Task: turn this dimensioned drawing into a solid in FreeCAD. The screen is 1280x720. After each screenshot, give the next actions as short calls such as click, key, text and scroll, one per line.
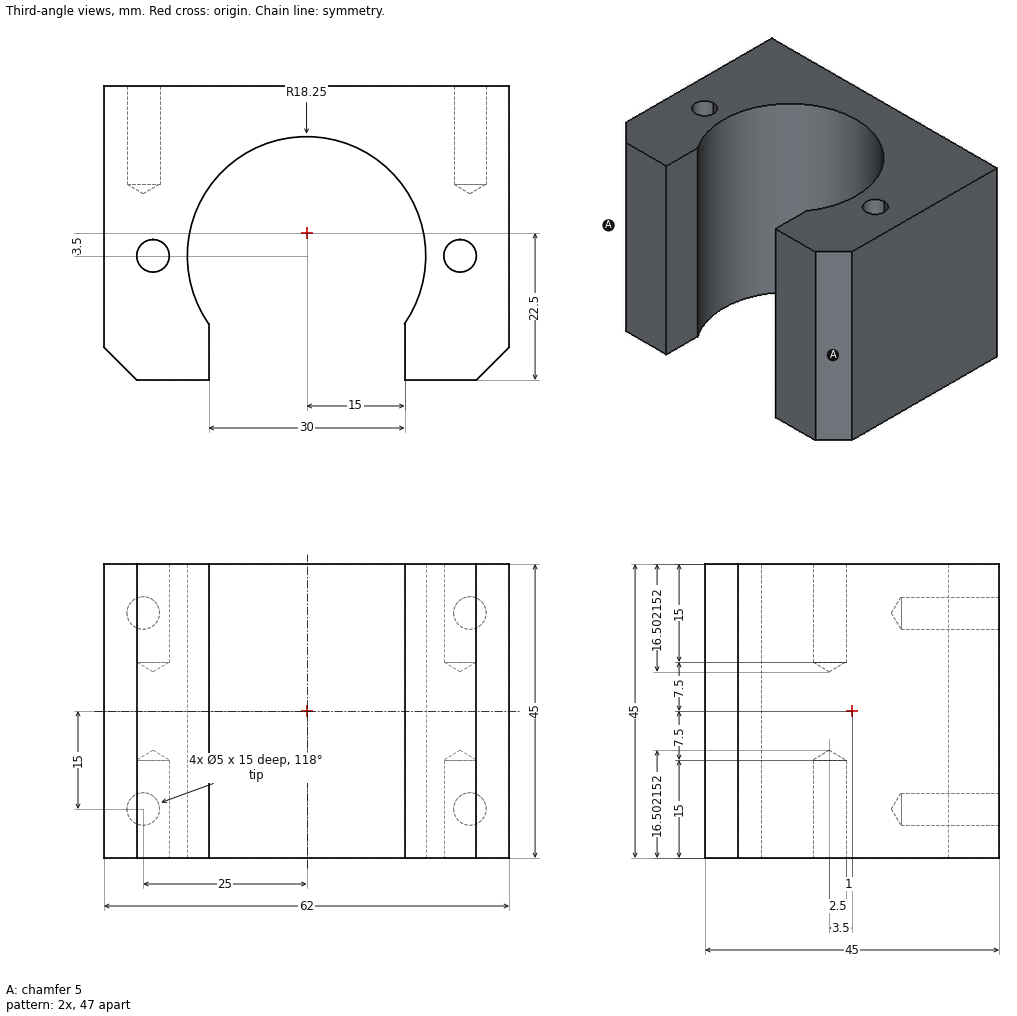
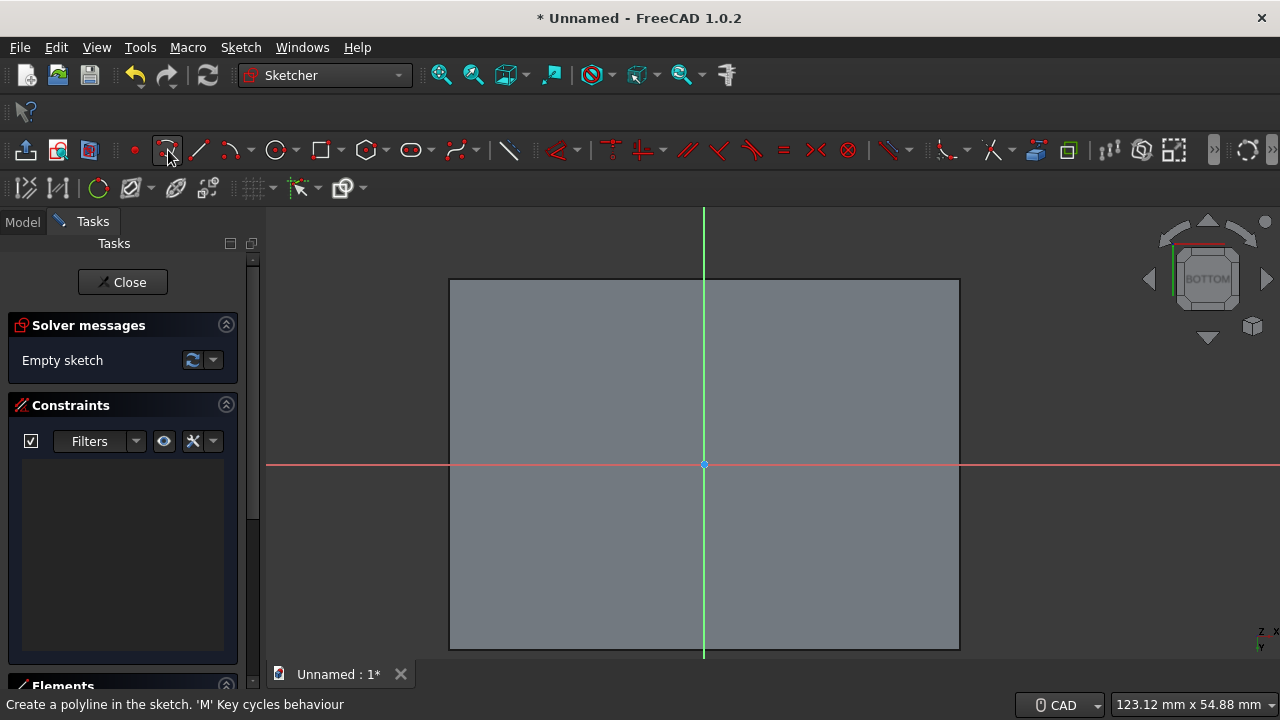
click(828, 350)
click(828, 279)
click(581, 279)
click(581, 350)
right_click(581, 350)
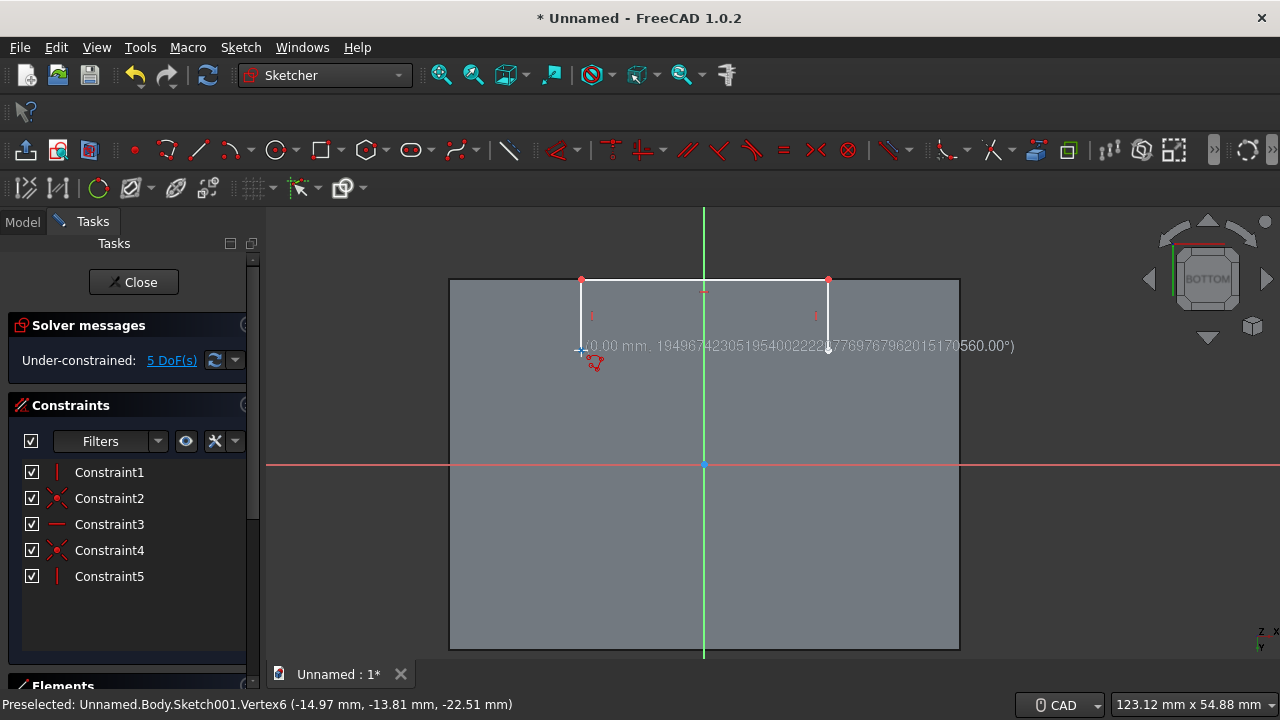
key(g)
key(3)
key(a)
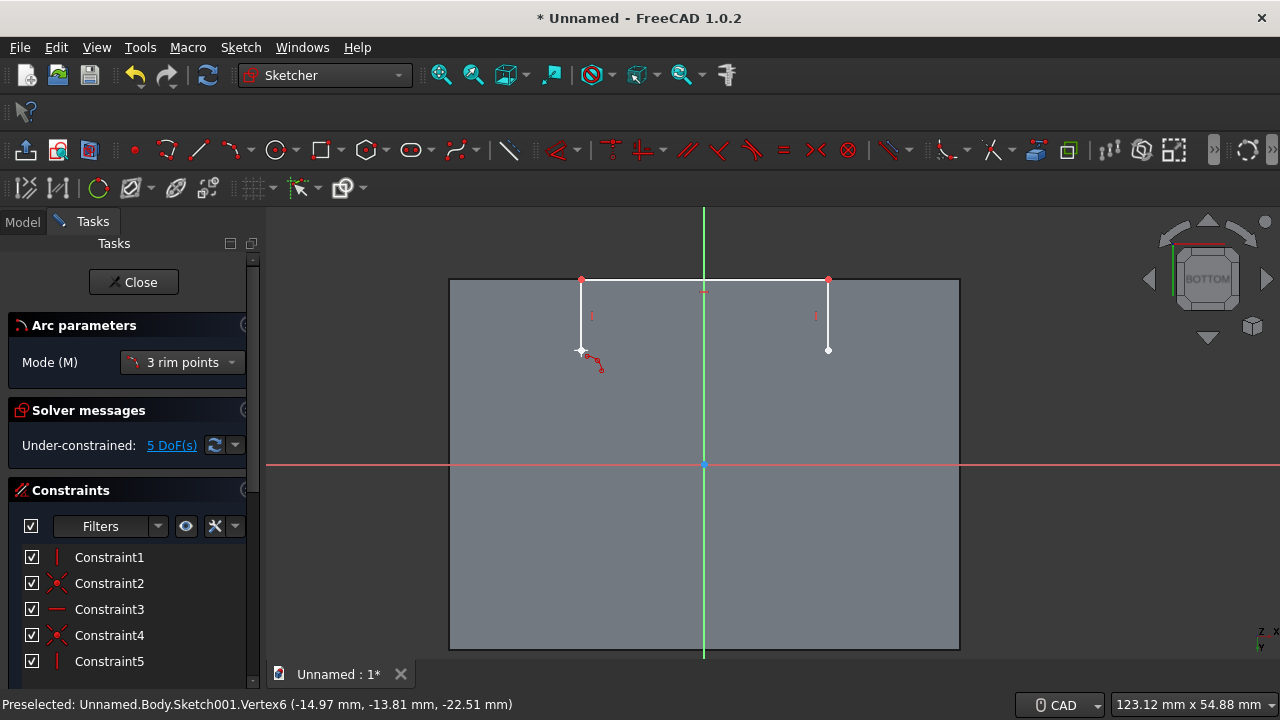
click(581, 351)
click(828, 351)
click(641, 572)
key(Escape)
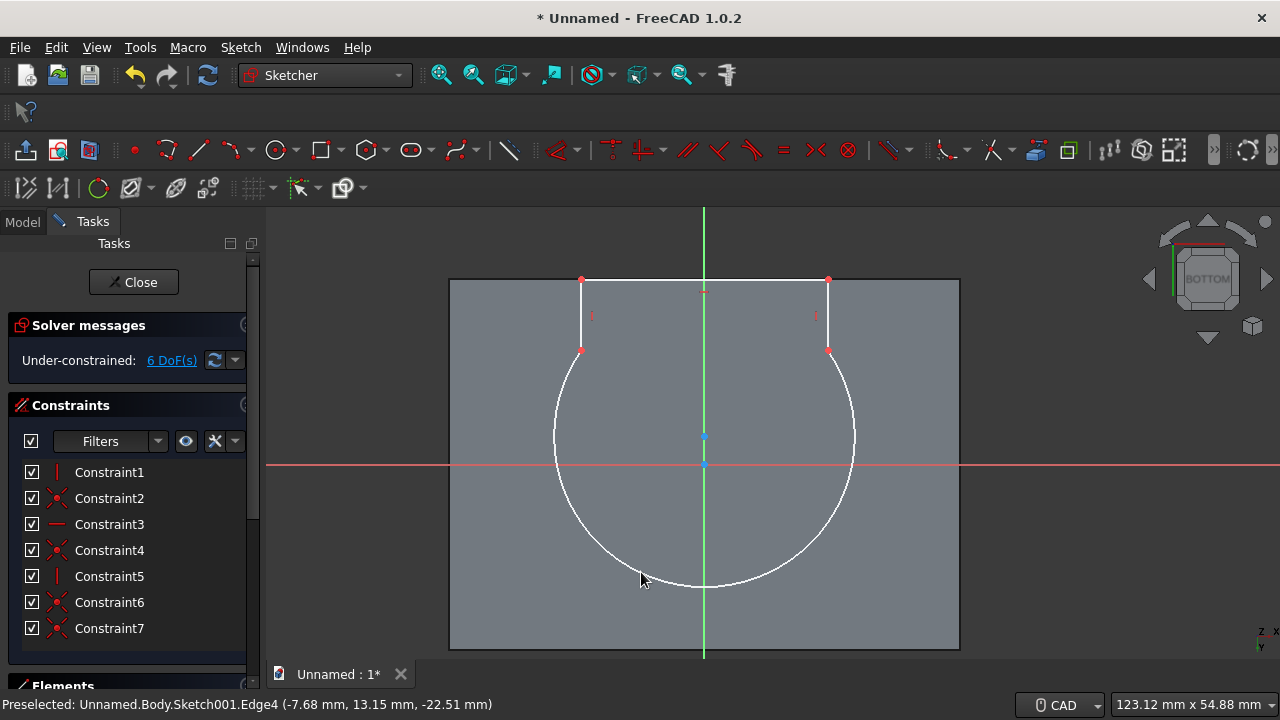
click(704, 437)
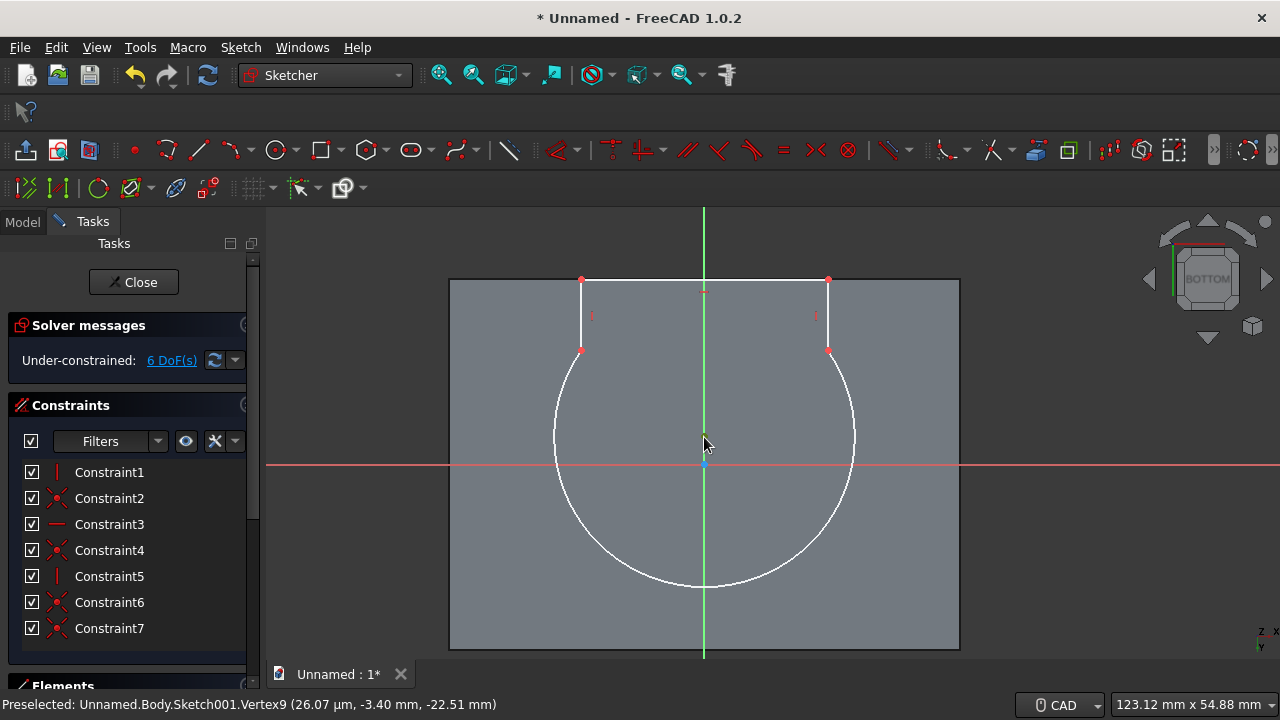
click(704, 546)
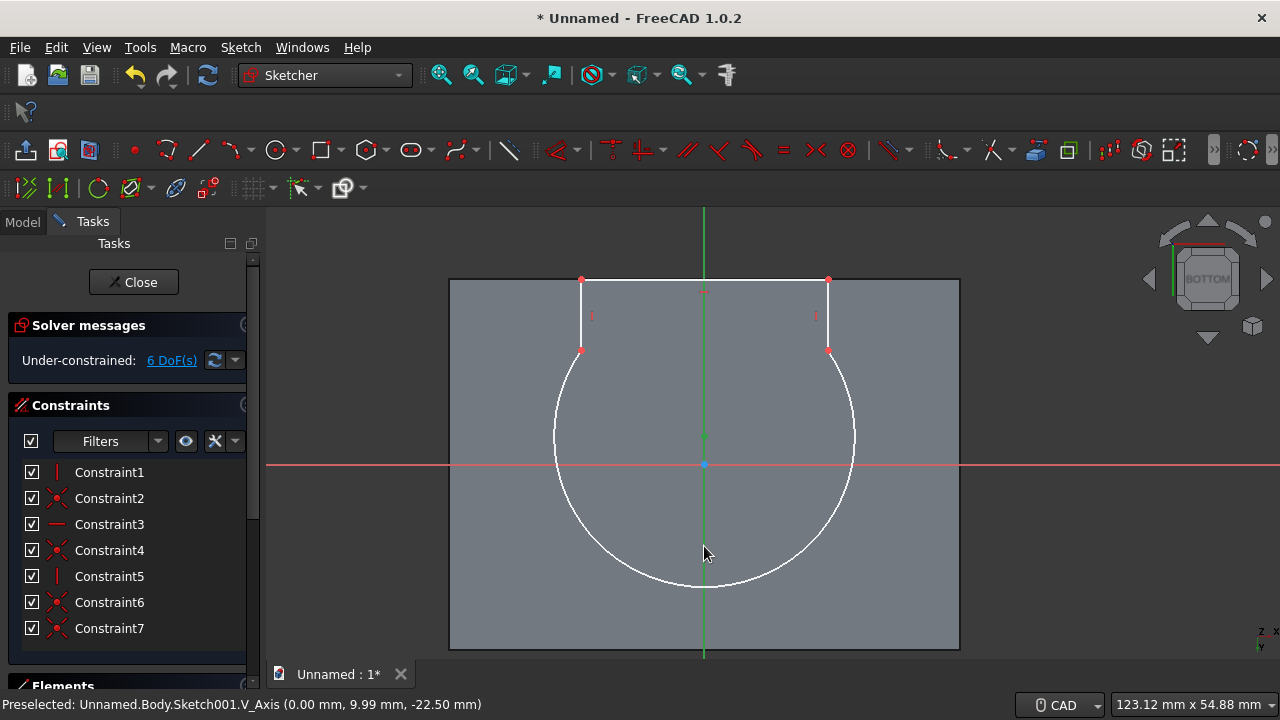
click(612, 150)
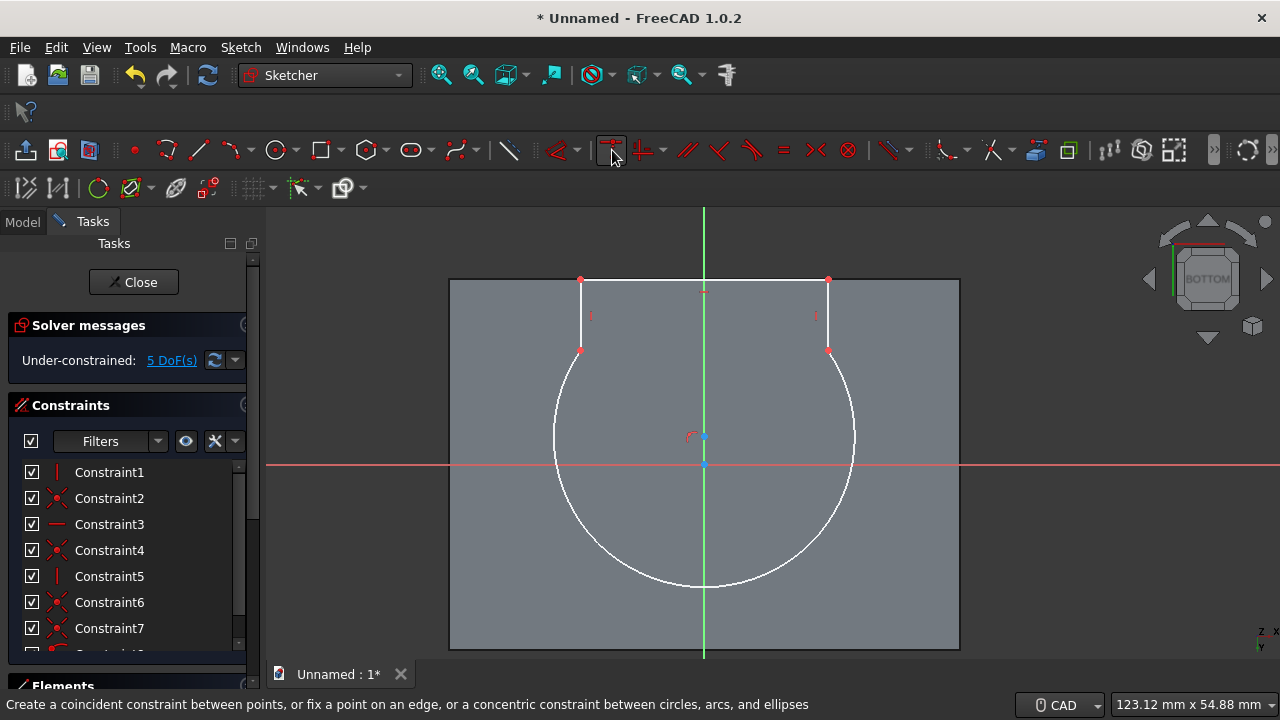
click(556, 150)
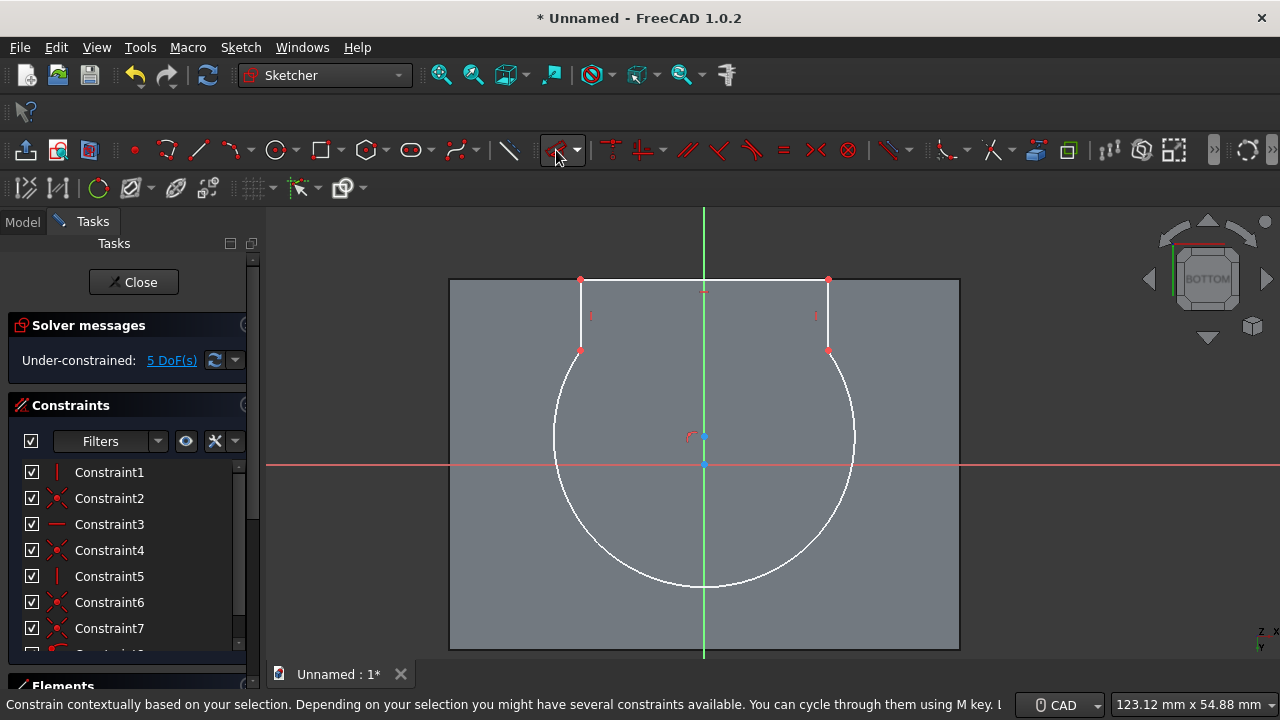
click(589, 534)
click(565, 555)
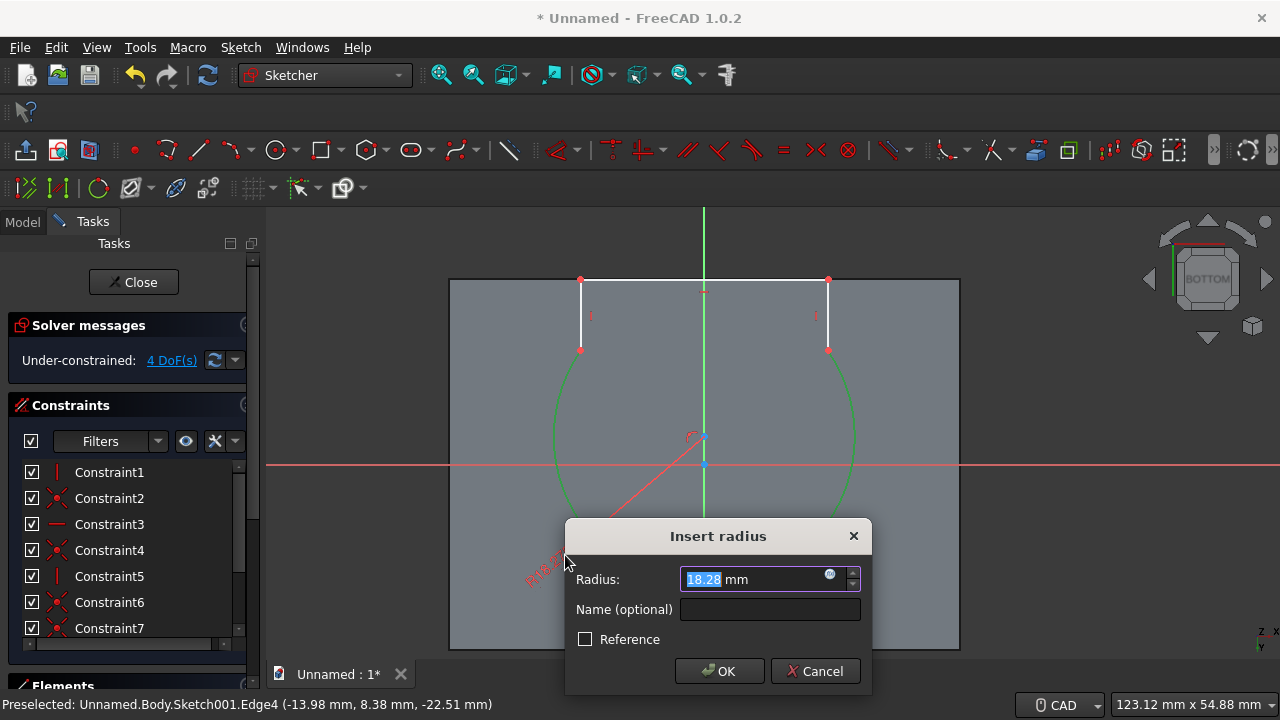
text(18.25)
key(Return)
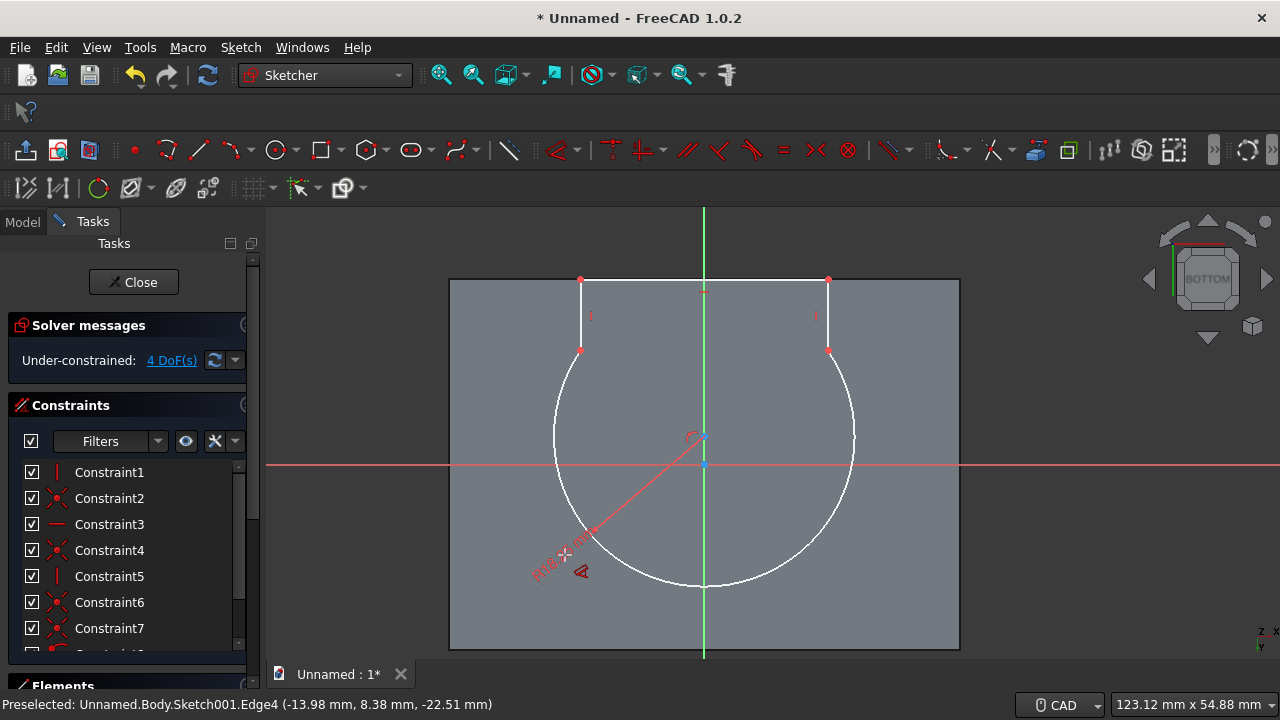
click(754, 280)
click(647, 246)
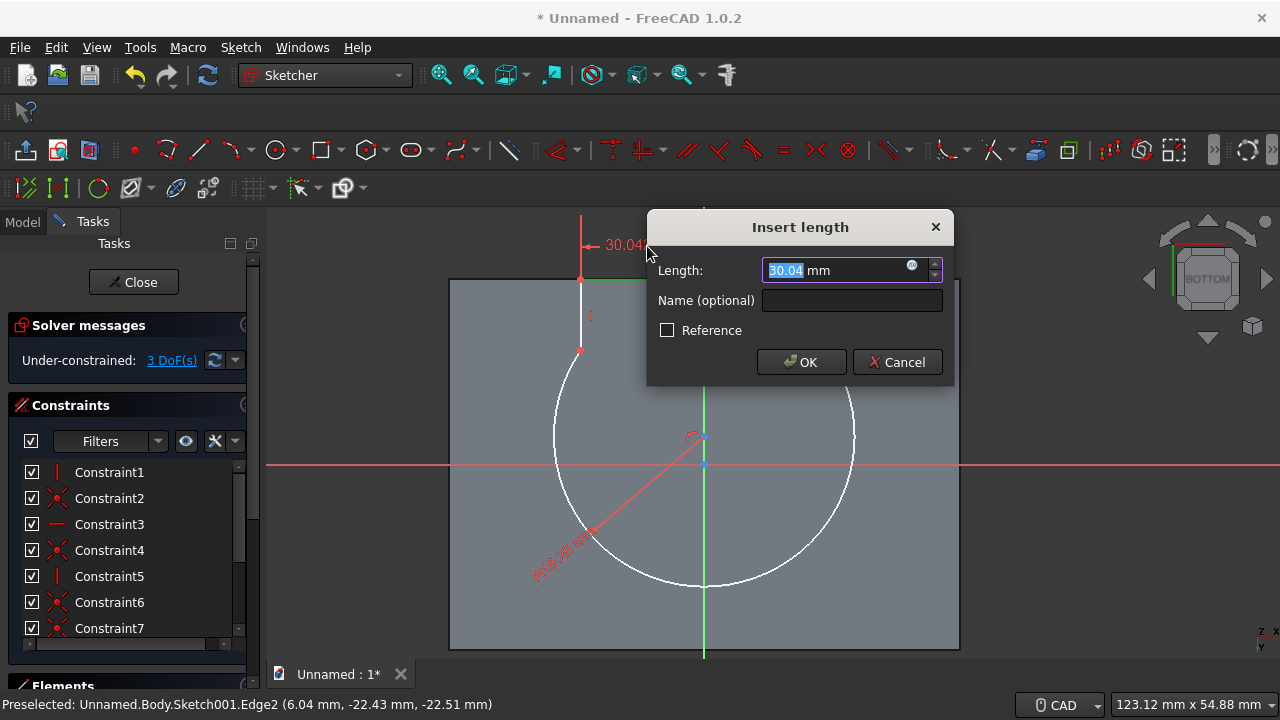
text(30)
key(Return)